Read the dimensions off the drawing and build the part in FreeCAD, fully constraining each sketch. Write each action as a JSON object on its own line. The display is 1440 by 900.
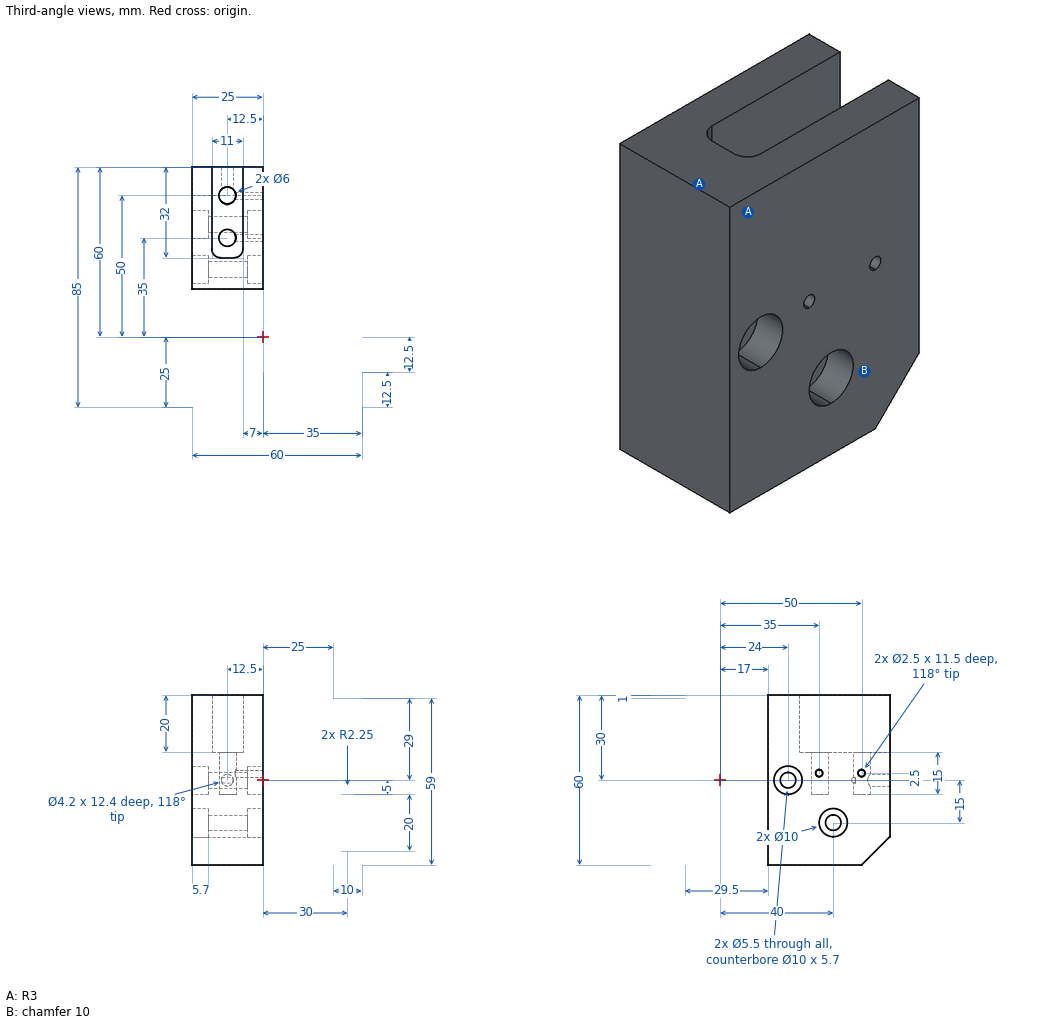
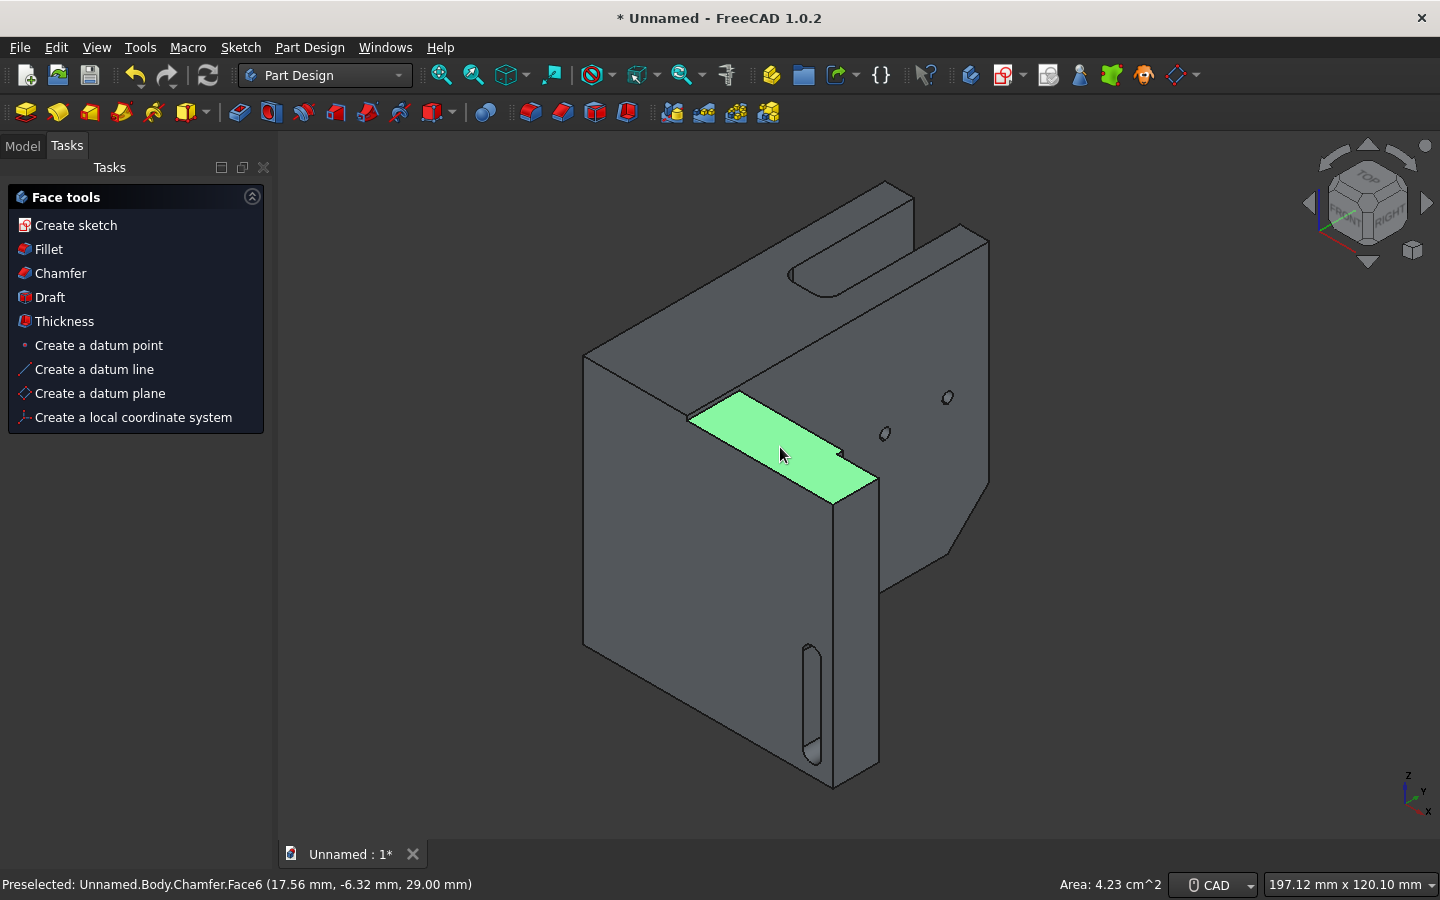
{"action": "left_click", "coordinate": [1004, 76]}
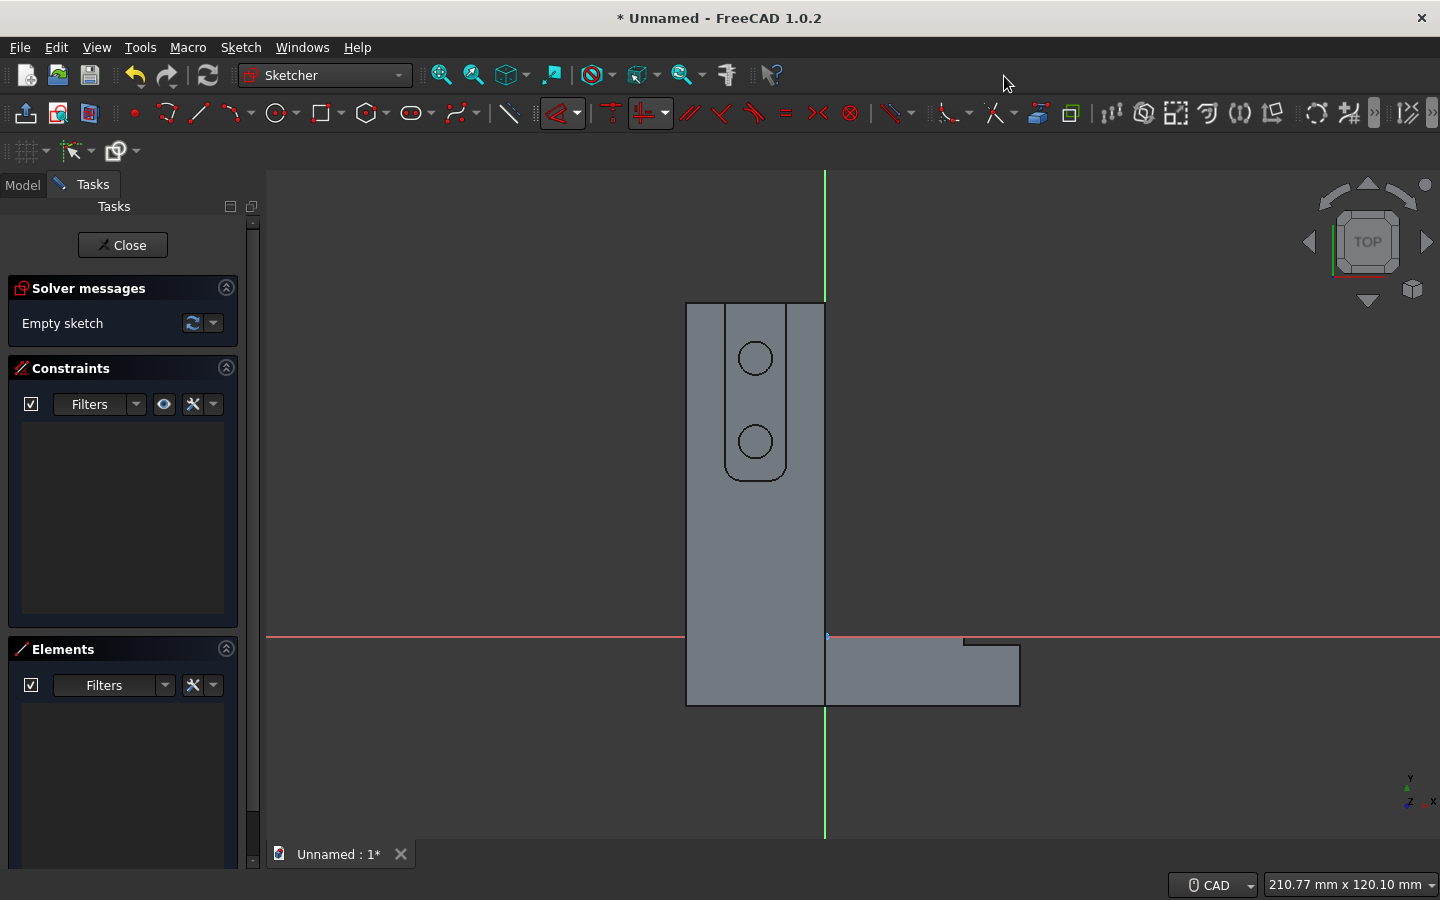
{"action": "left_click", "coordinate": [90, 114]}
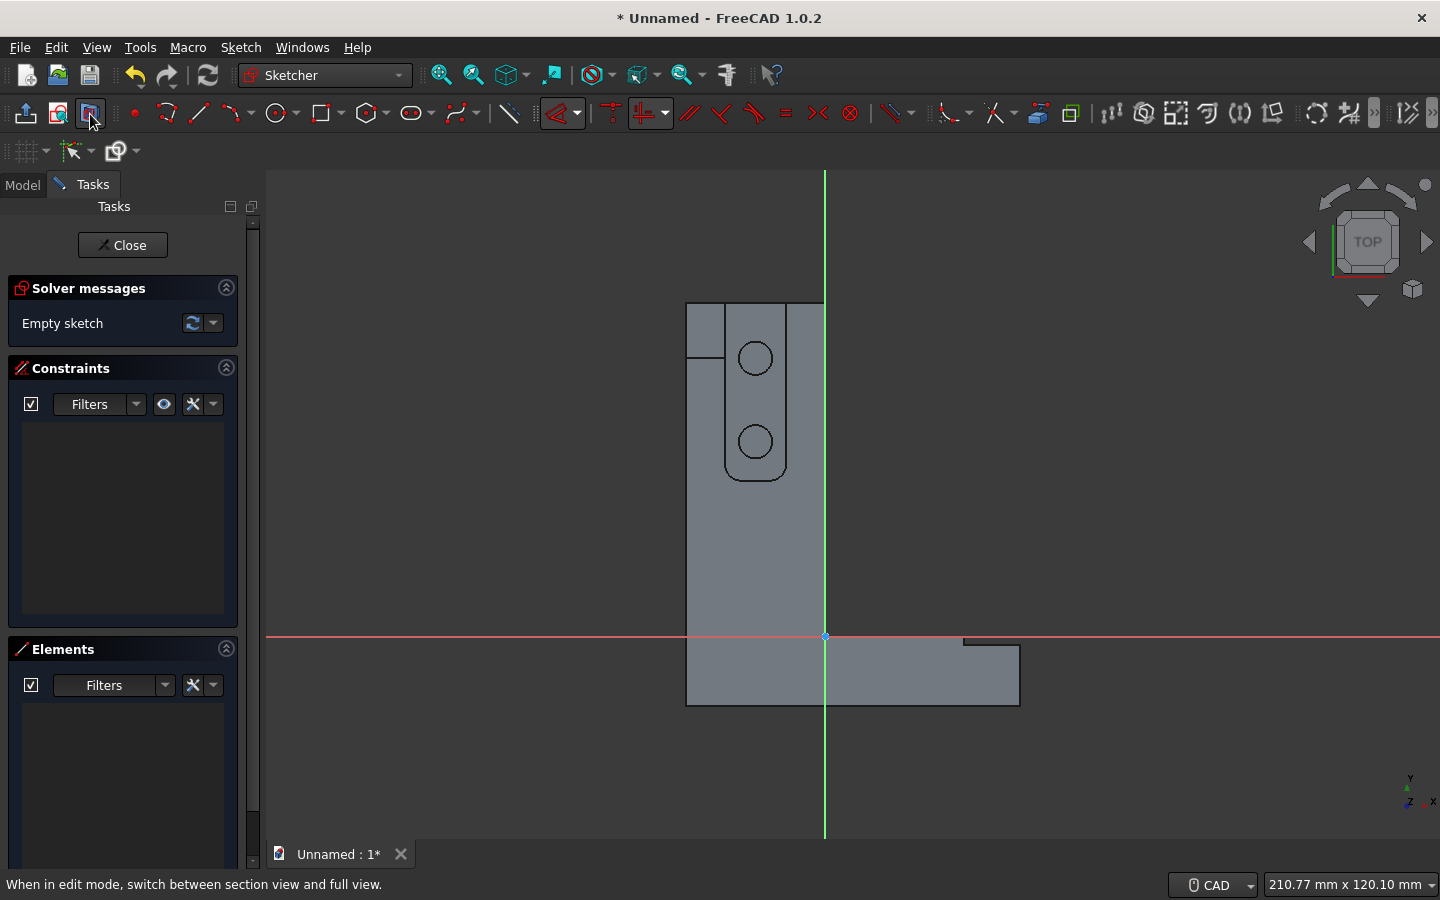
{"action": "scroll", "coordinate": [982, 744], "scroll_direction": "up", "scroll_amount": 6}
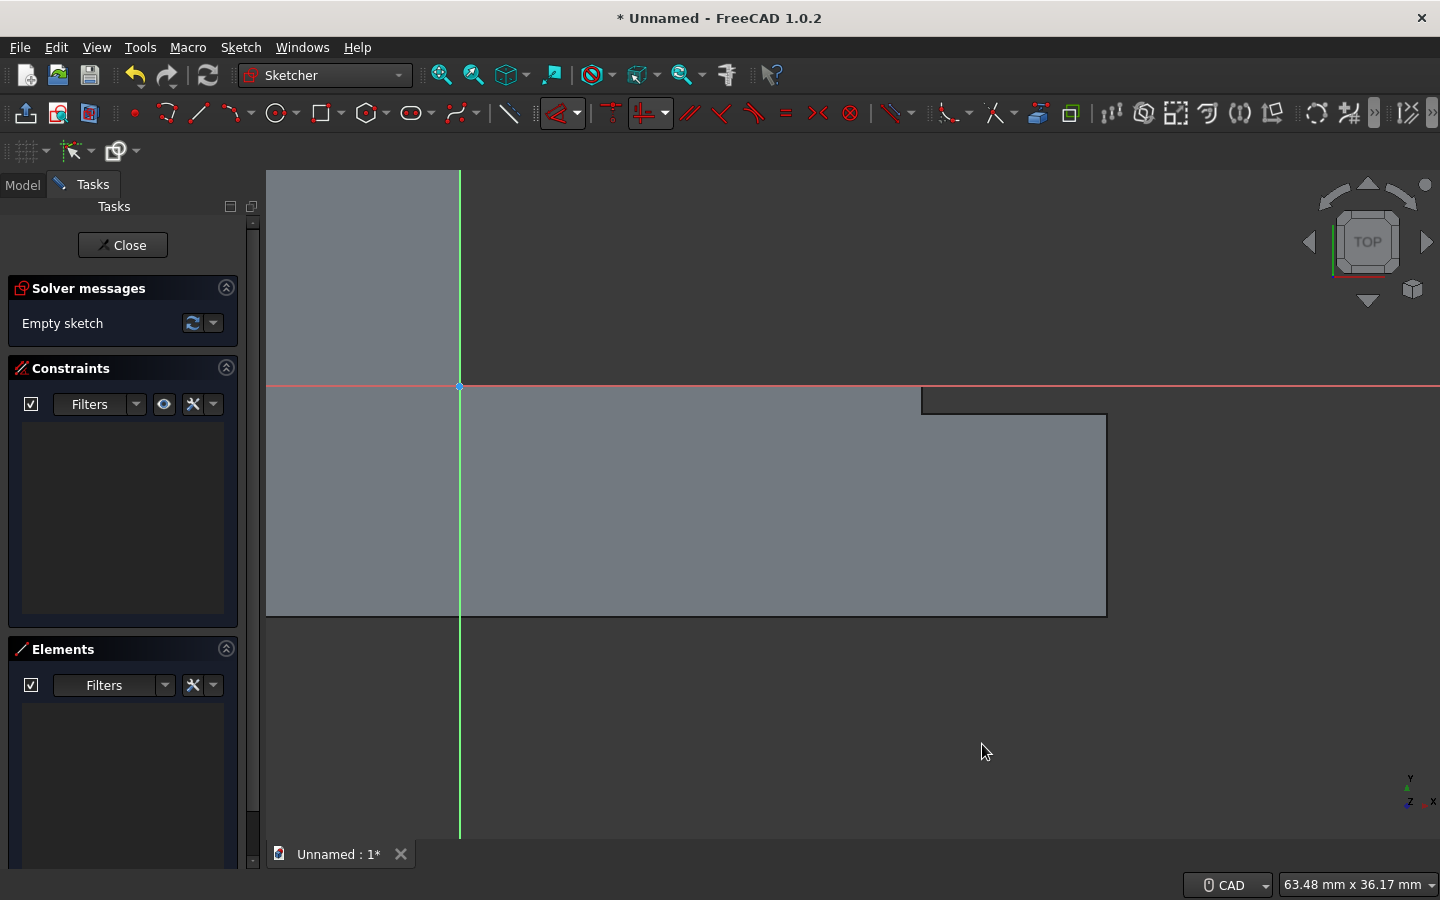
{"action": "left_click", "coordinate": [322, 114]}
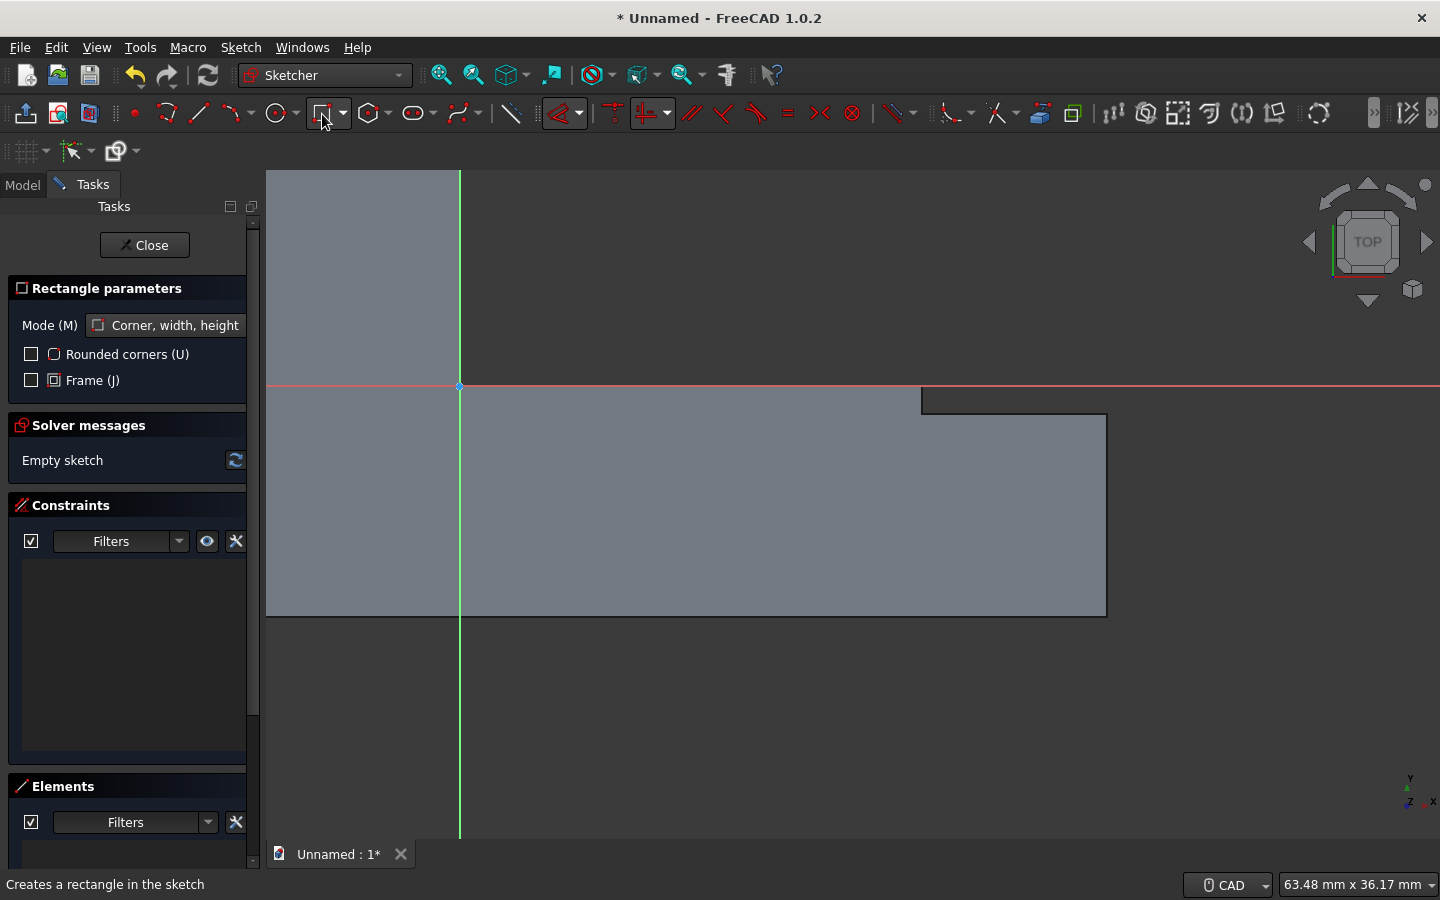
{"action": "left_click", "coordinate": [460, 386]}
{"action": "mouse_move", "coordinate": [1107, 617]}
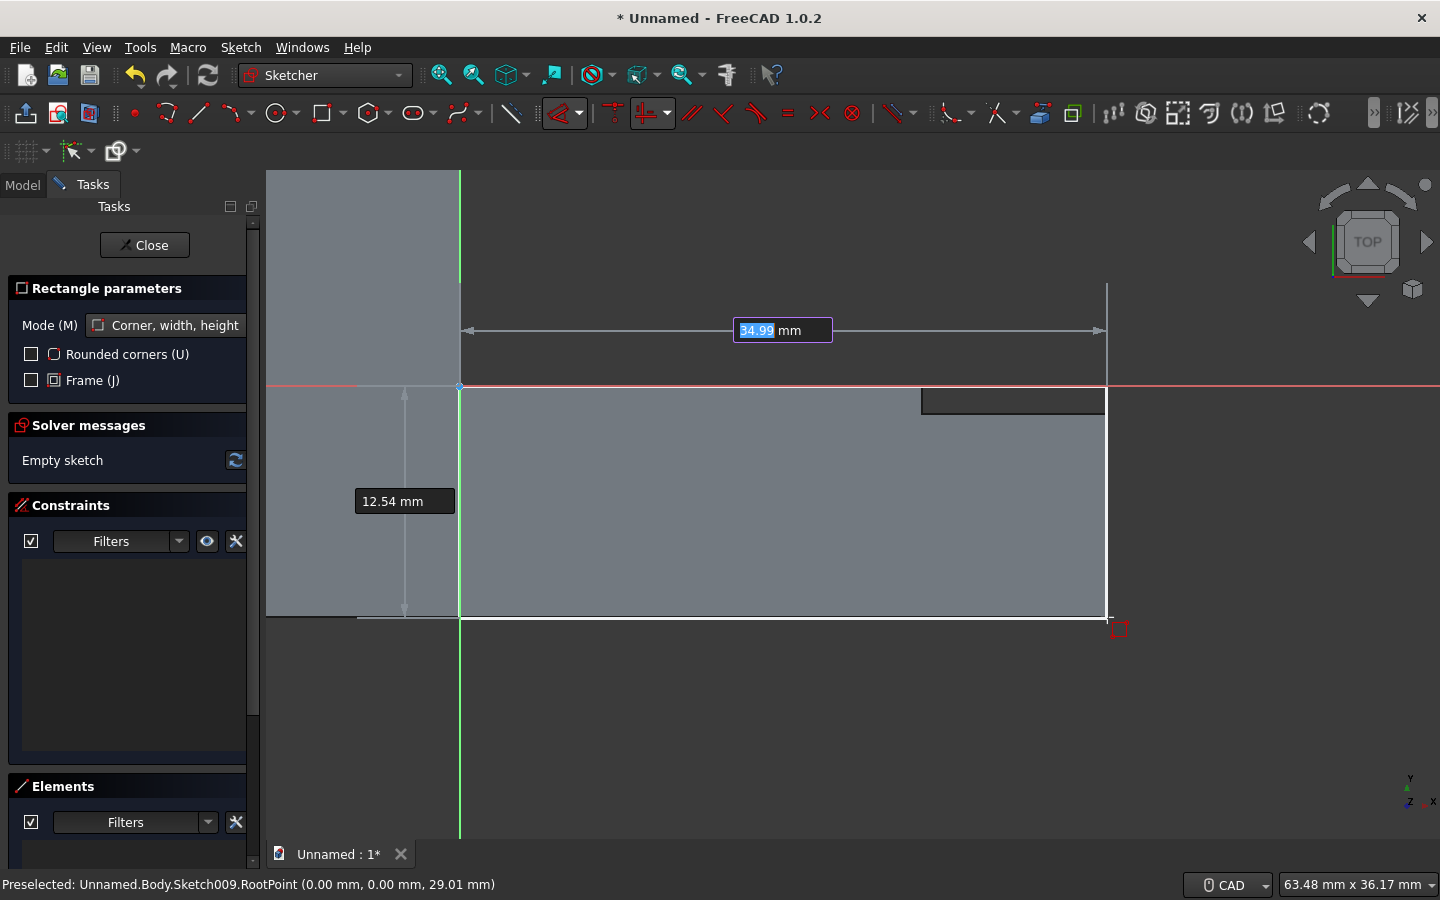
{"action": "type", "text": "35"}
{"action": "key", "text": "Tab"}
{"action": "type", "text": "12.5"}
{"action": "key", "text": "Return"}
{"action": "key", "text": "Escape"}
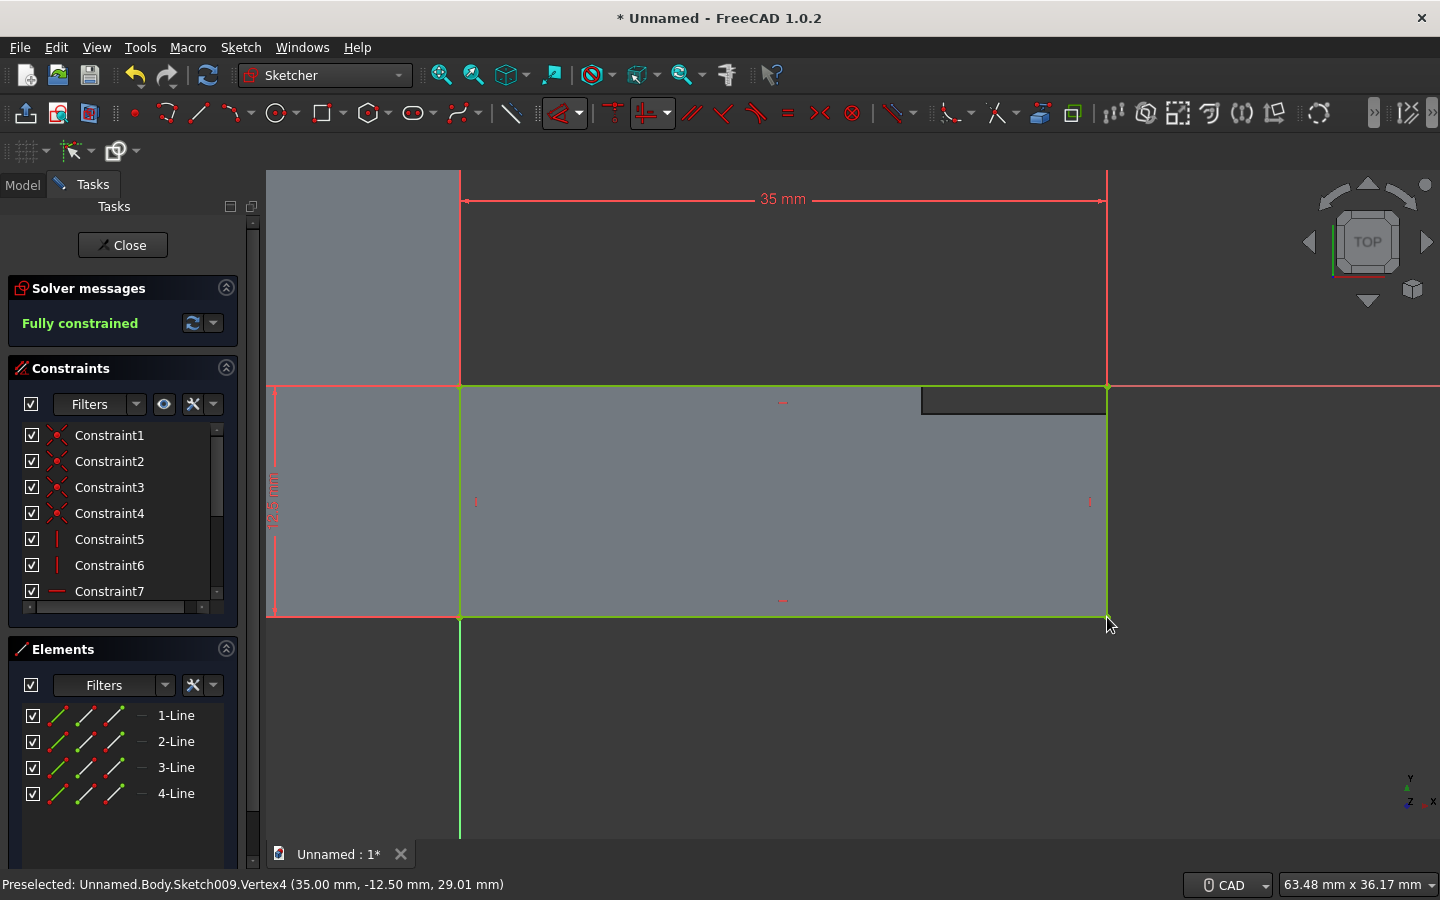
{"action": "left_click", "coordinate": [123, 245]}